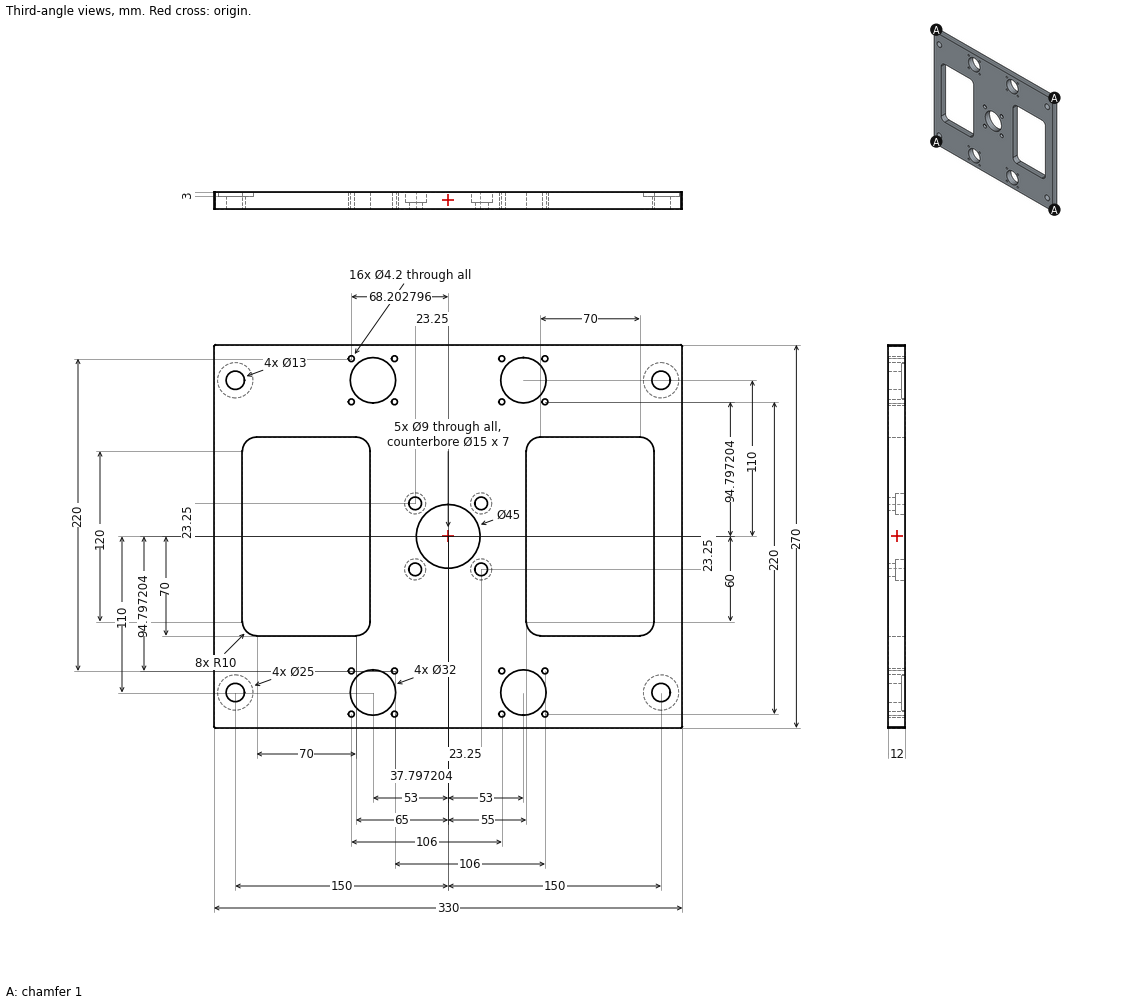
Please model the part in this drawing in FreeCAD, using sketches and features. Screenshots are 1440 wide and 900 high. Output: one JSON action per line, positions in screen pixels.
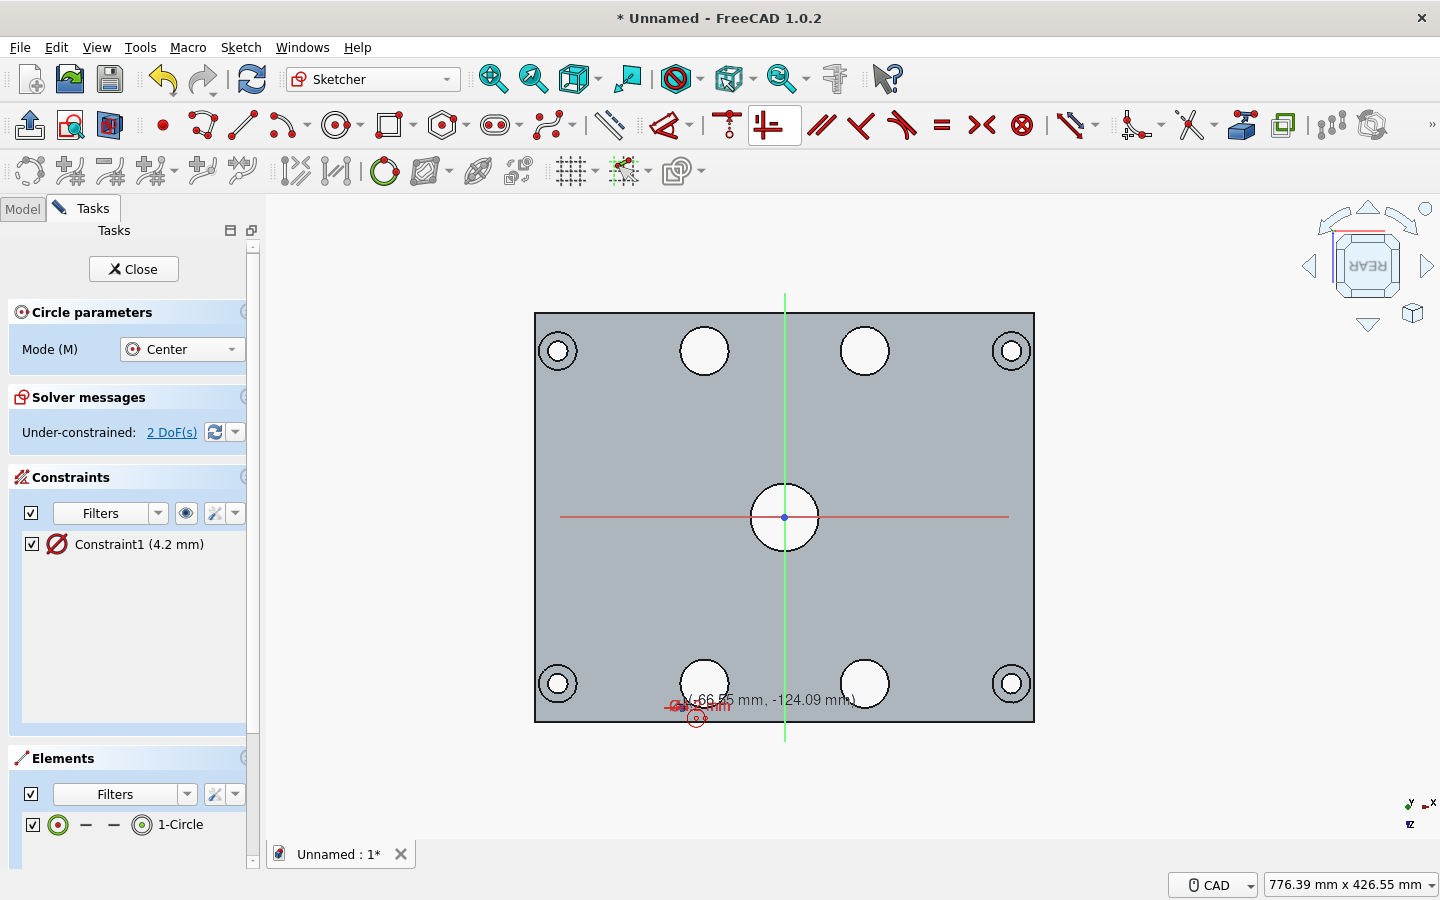
{"action": "scroll", "coordinate": [682, 328], "scroll_direction": "up", "scroll_amount": 10}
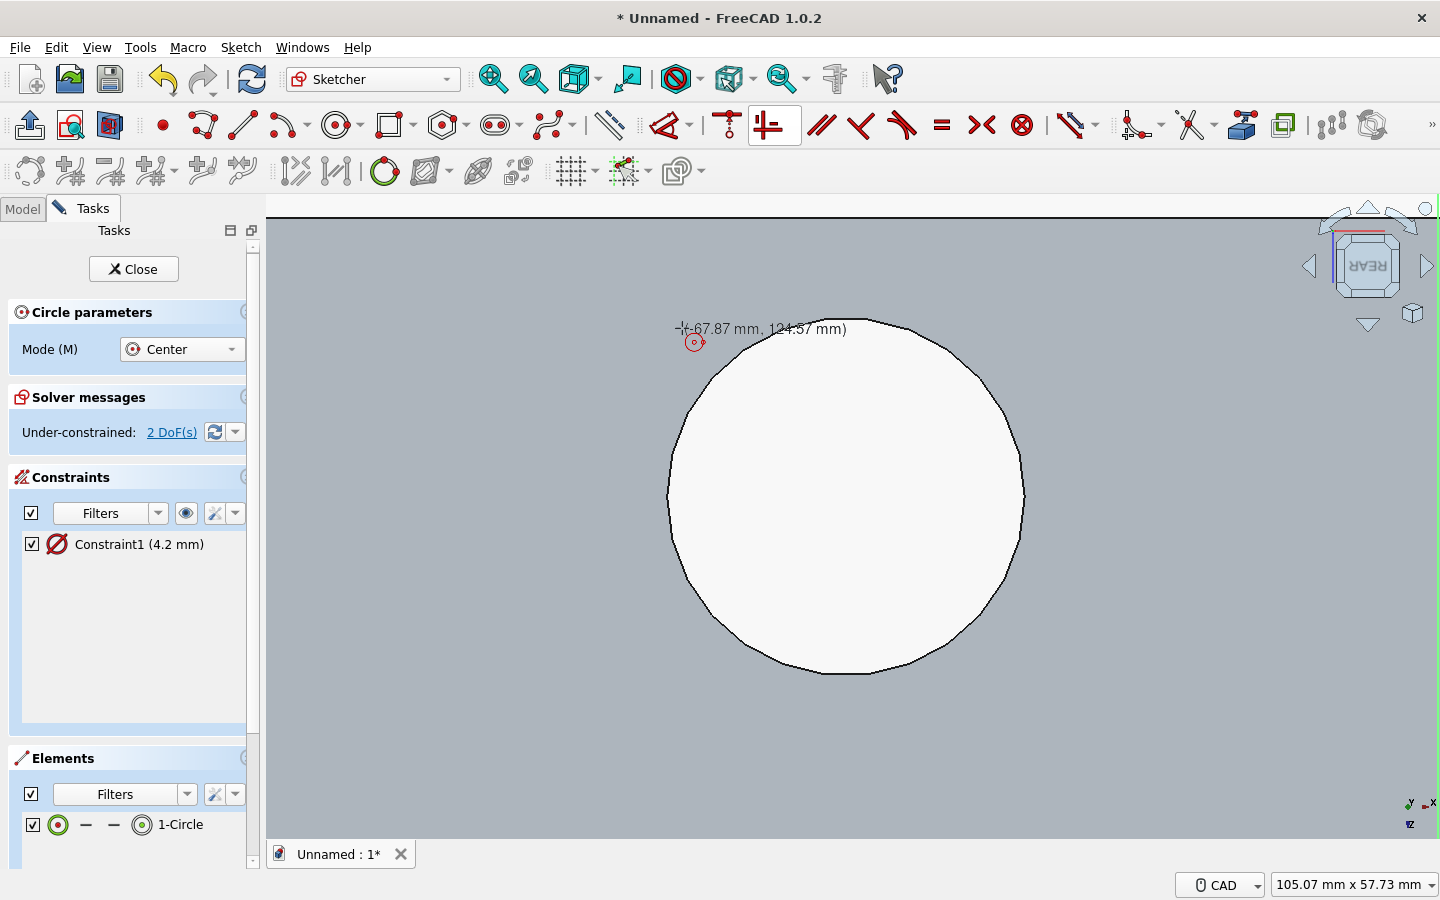
{"action": "scroll", "coordinate": [682, 327], "scroll_direction": "down", "scroll_amount": 10}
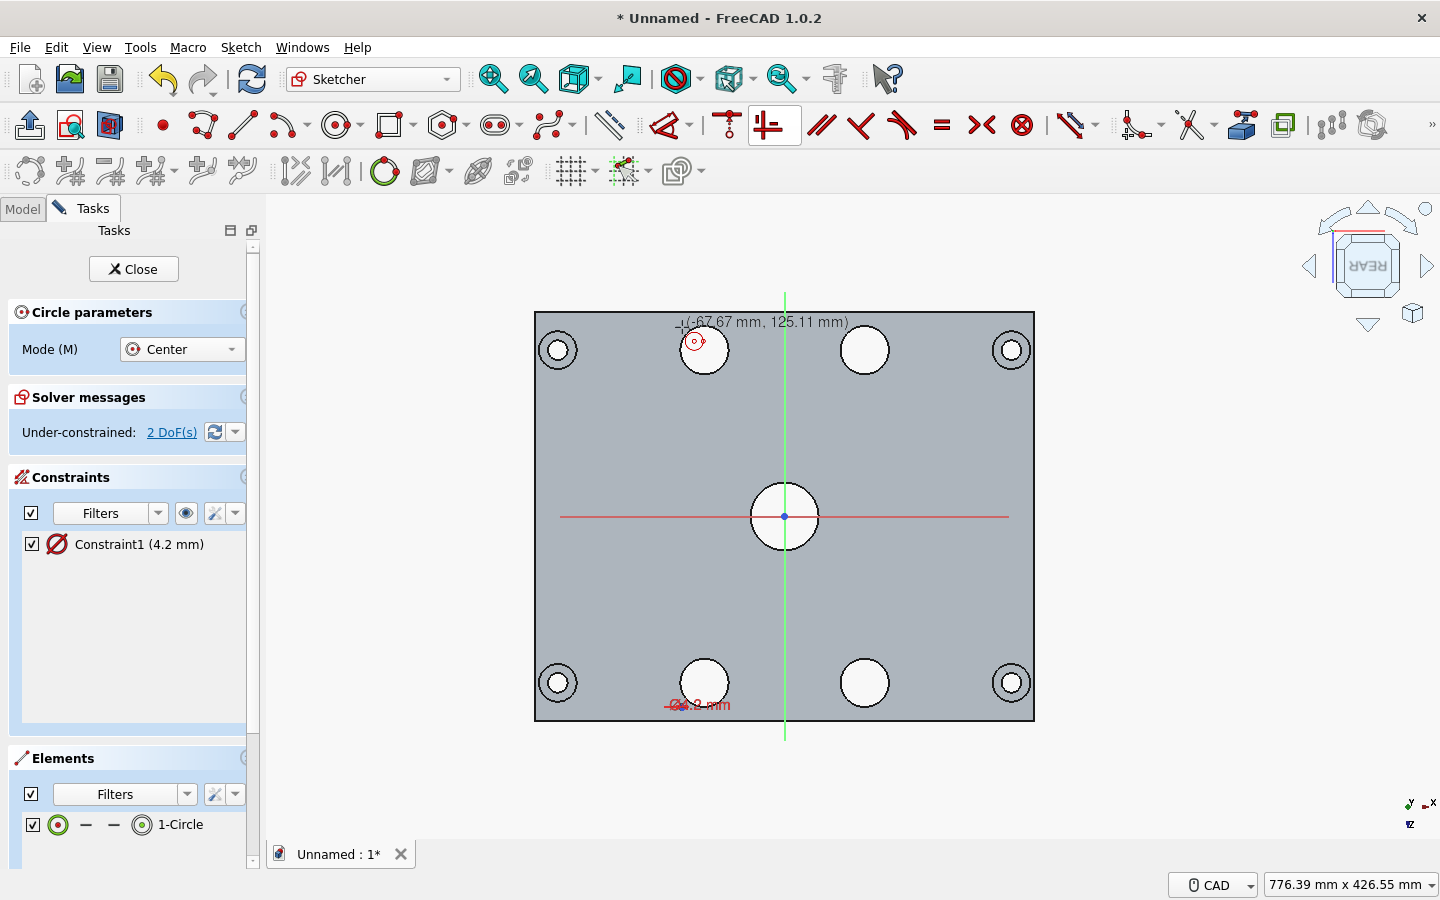
{"action": "left_click", "coordinate": [682, 327]}
{"action": "mouse_move", "coordinate": [684, 325]}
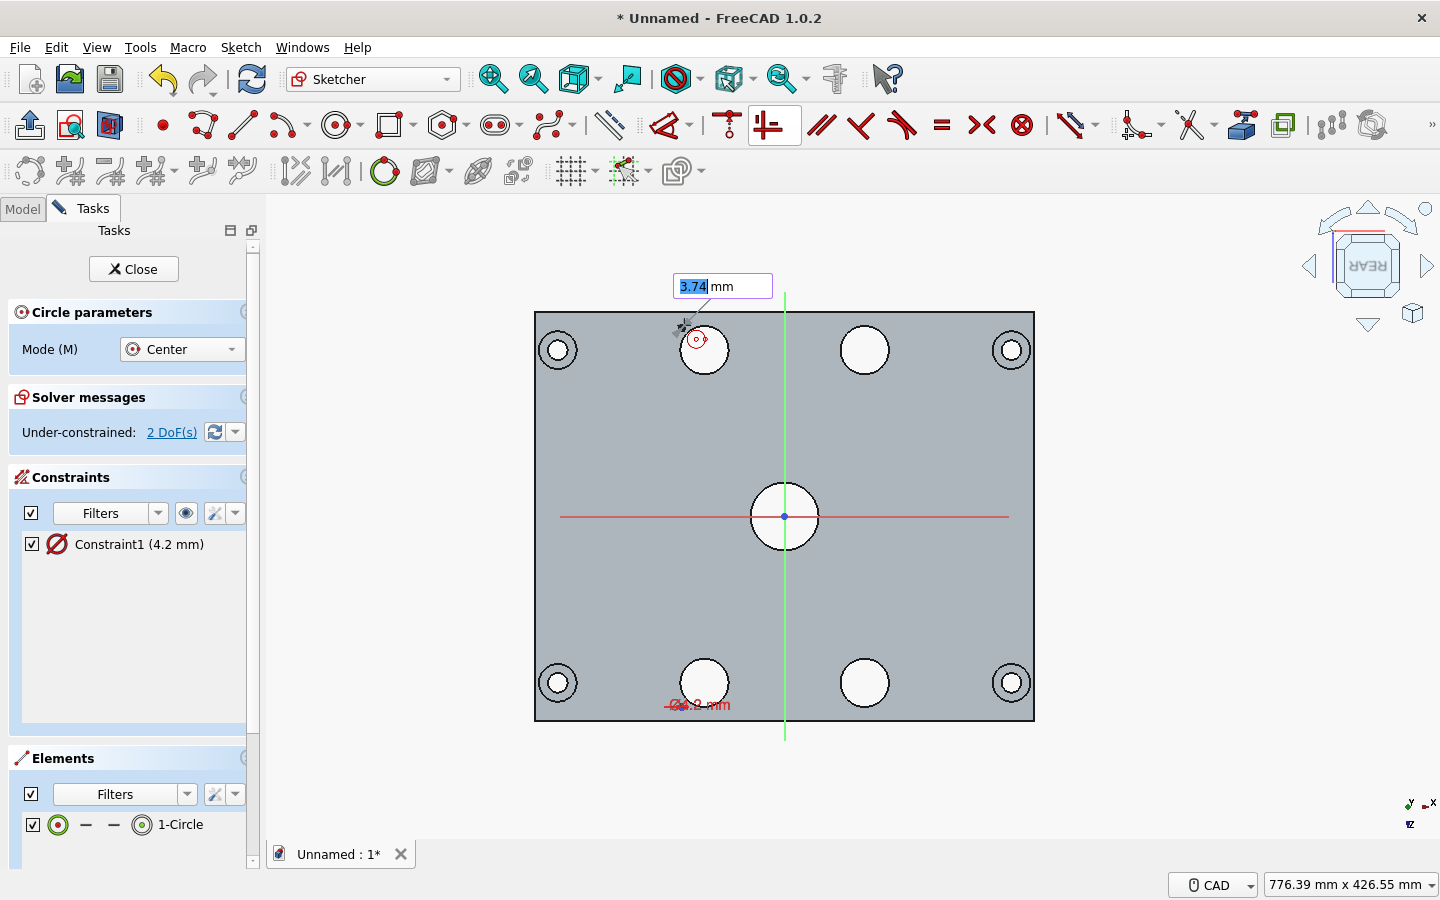
{"action": "type", "text": "4.2"}
{"action": "key", "text": "Return"}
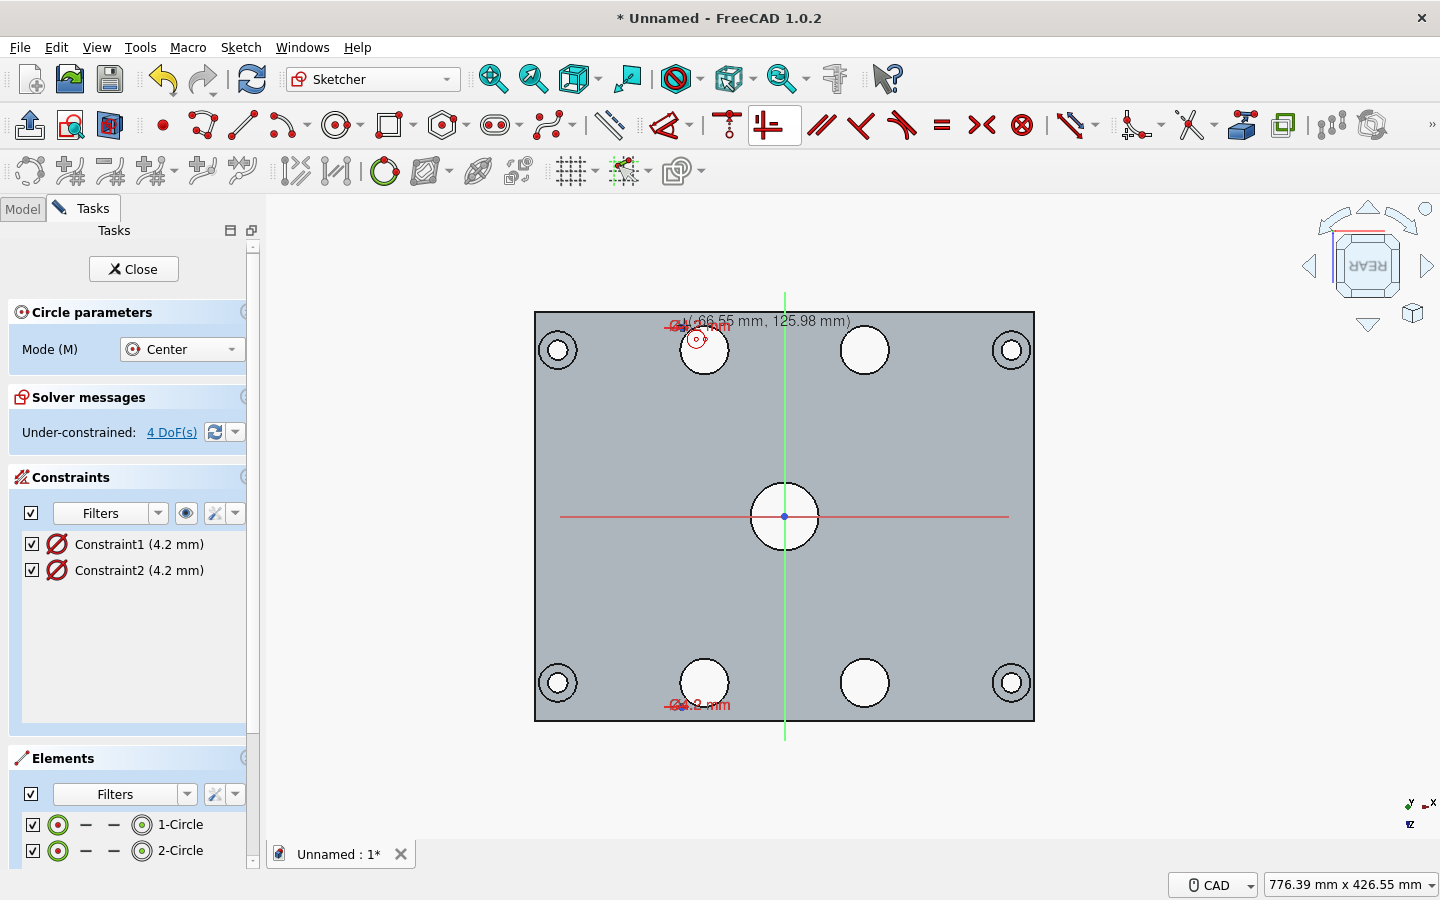
{"action": "scroll", "coordinate": [727, 327], "scroll_direction": "up", "scroll_amount": 10}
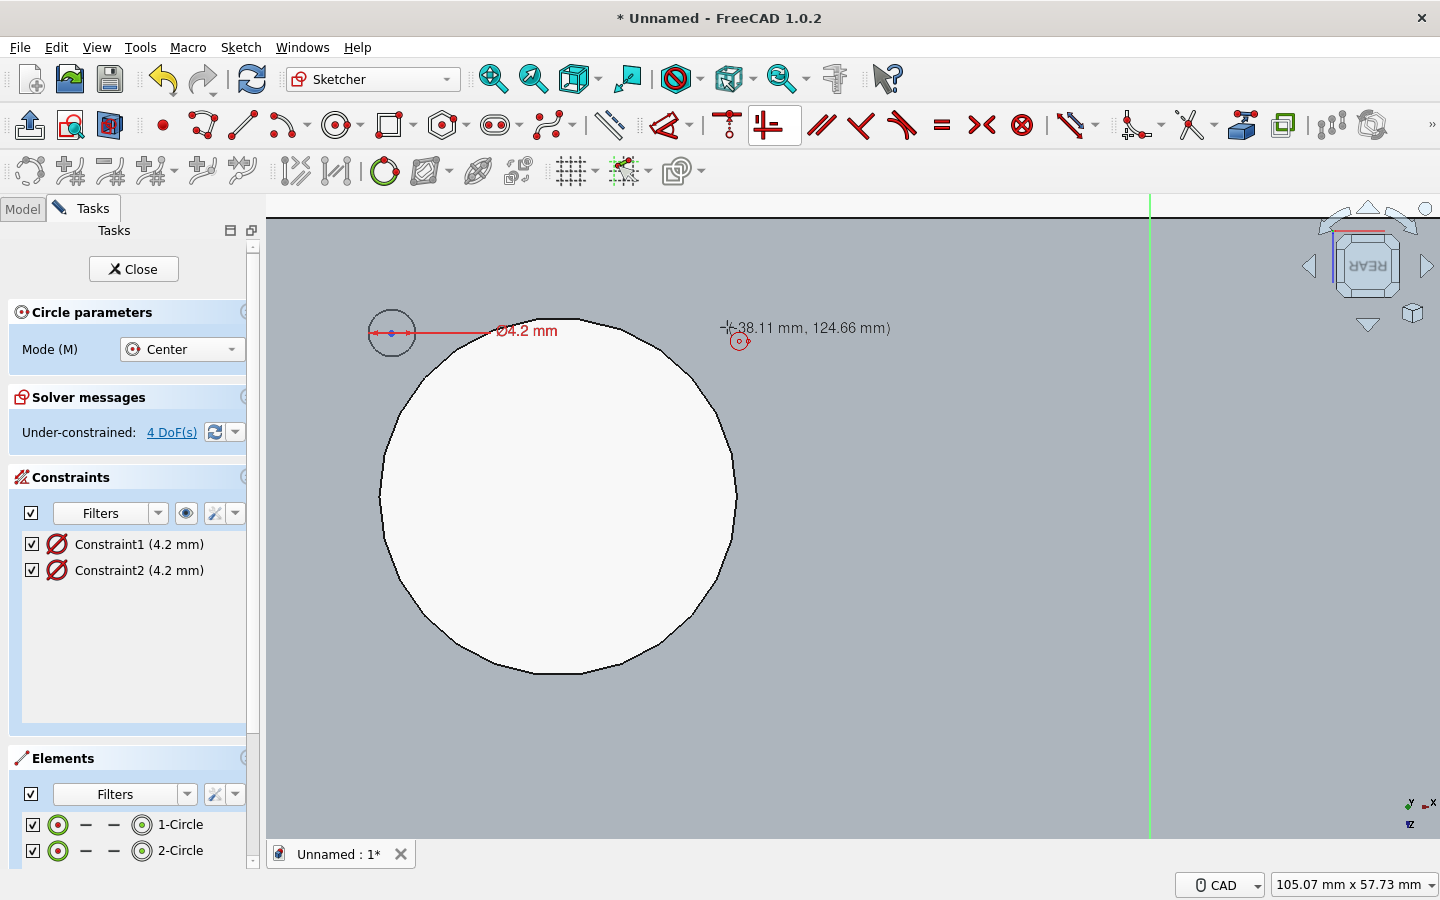
{"action": "scroll", "coordinate": [727, 327], "scroll_direction": "down", "scroll_amount": 10}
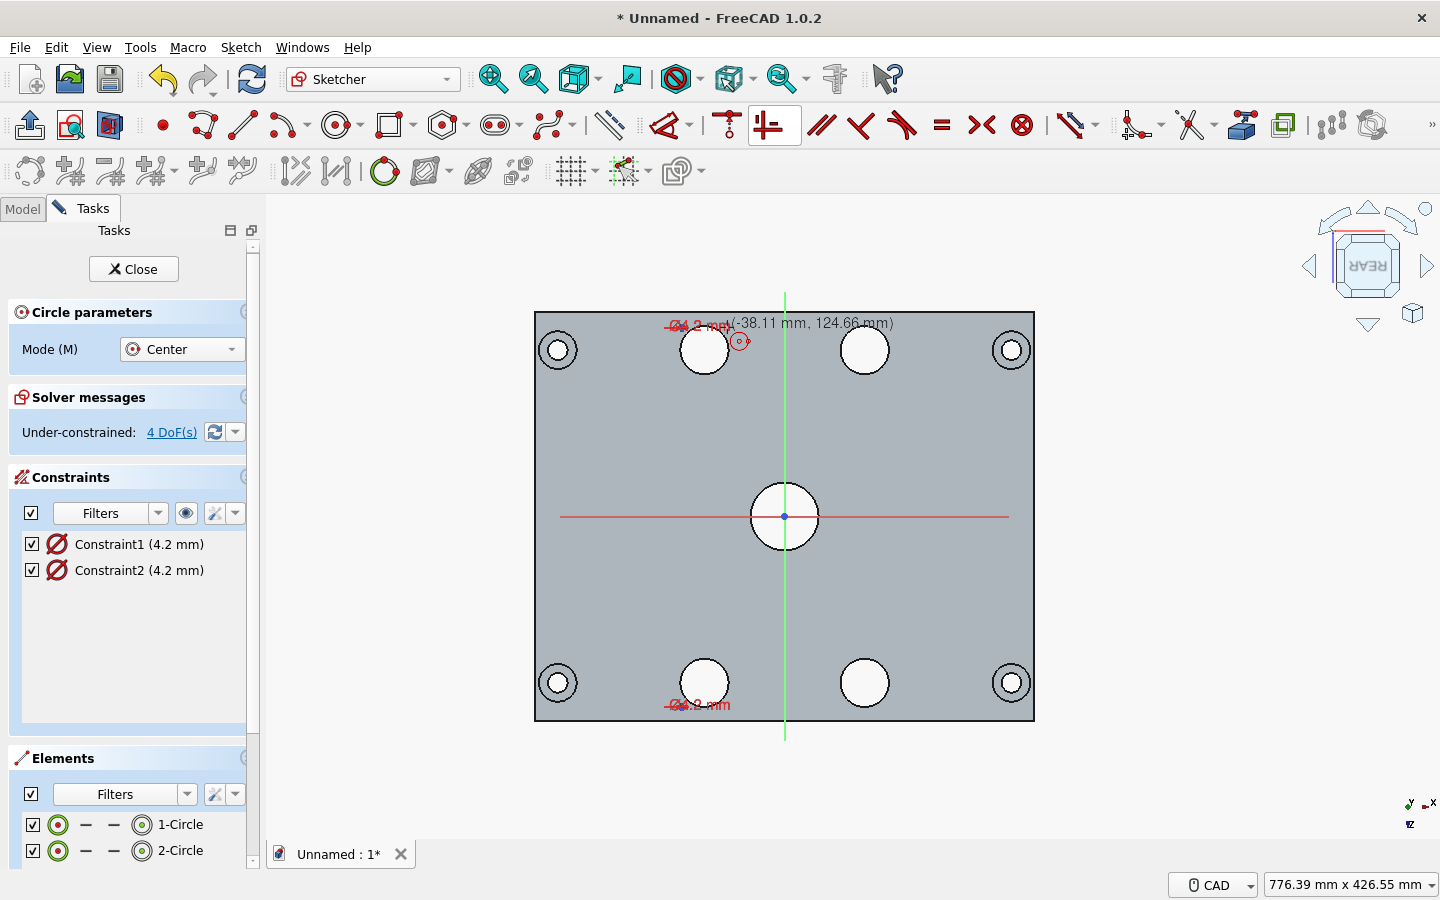
{"action": "left_click", "coordinate": [727, 327]}
{"action": "mouse_move", "coordinate": [730, 325]}